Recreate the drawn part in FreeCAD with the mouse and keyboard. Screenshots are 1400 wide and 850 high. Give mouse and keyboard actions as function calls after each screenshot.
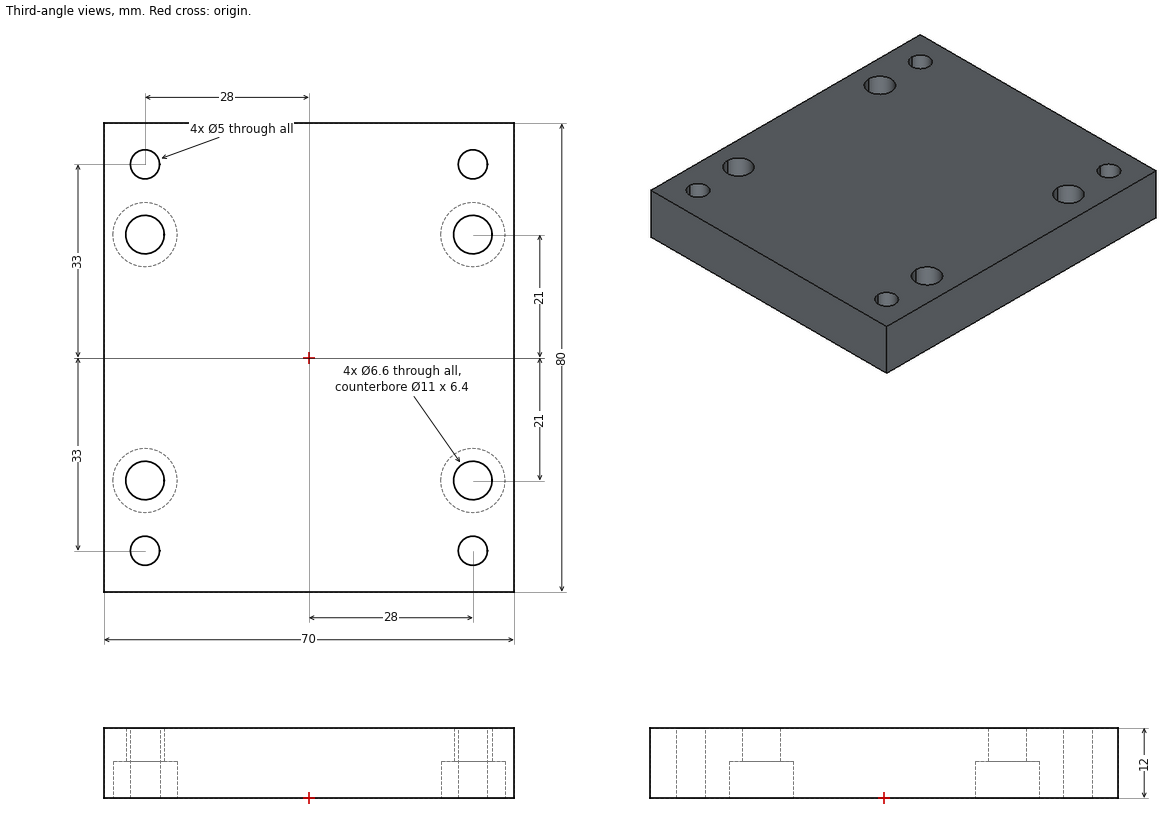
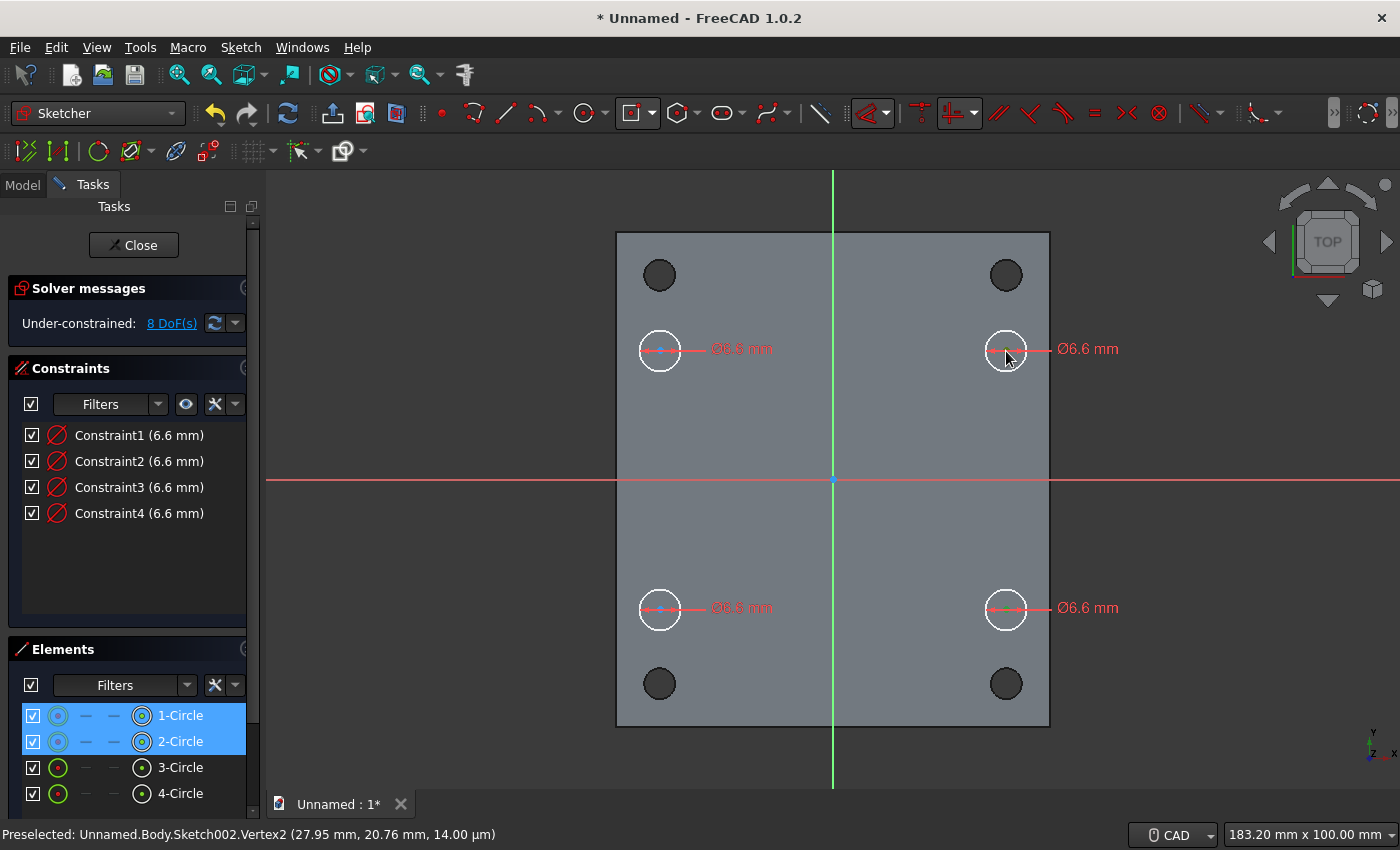
click(976, 114)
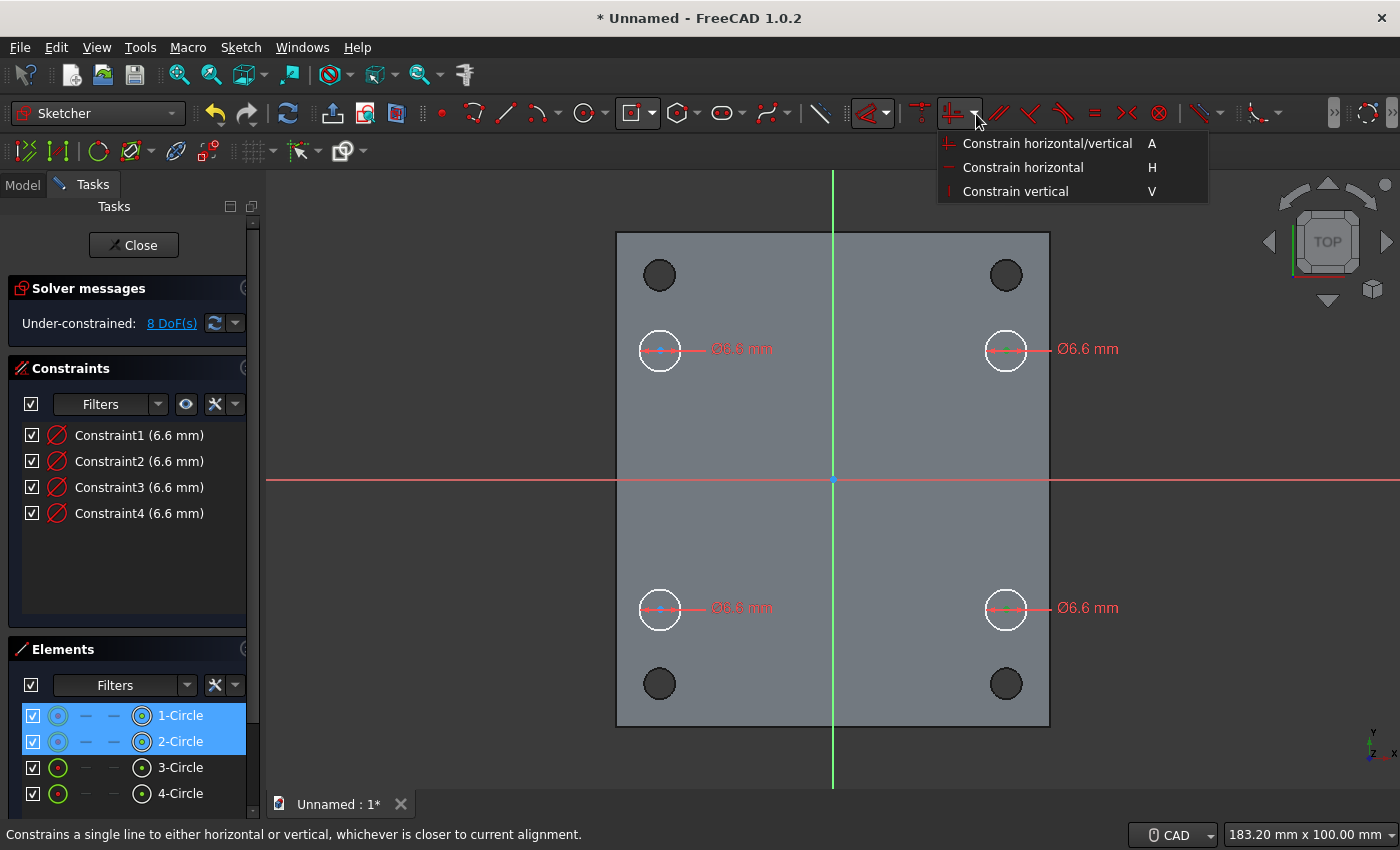
click(1073, 191)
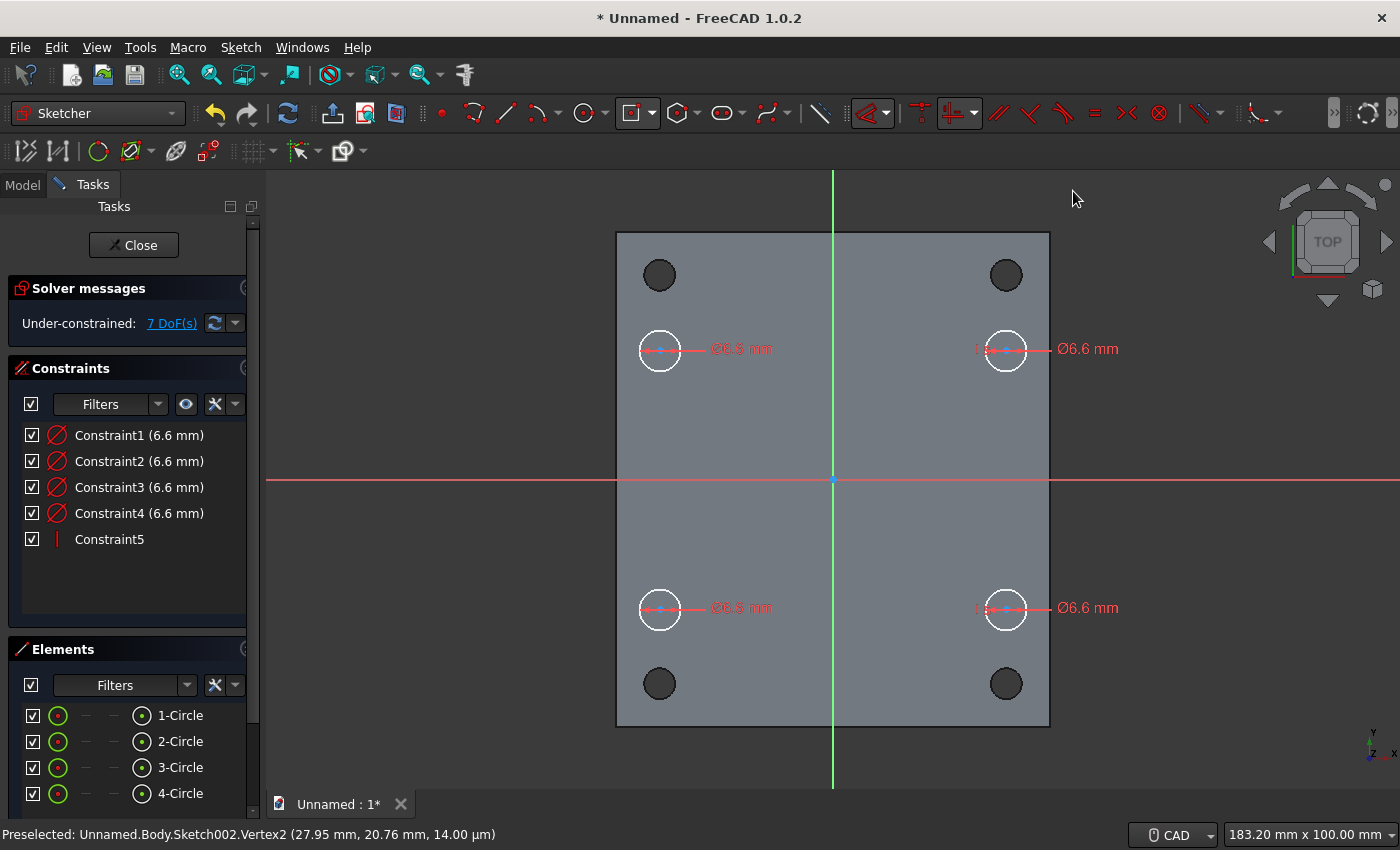
click(1006, 610)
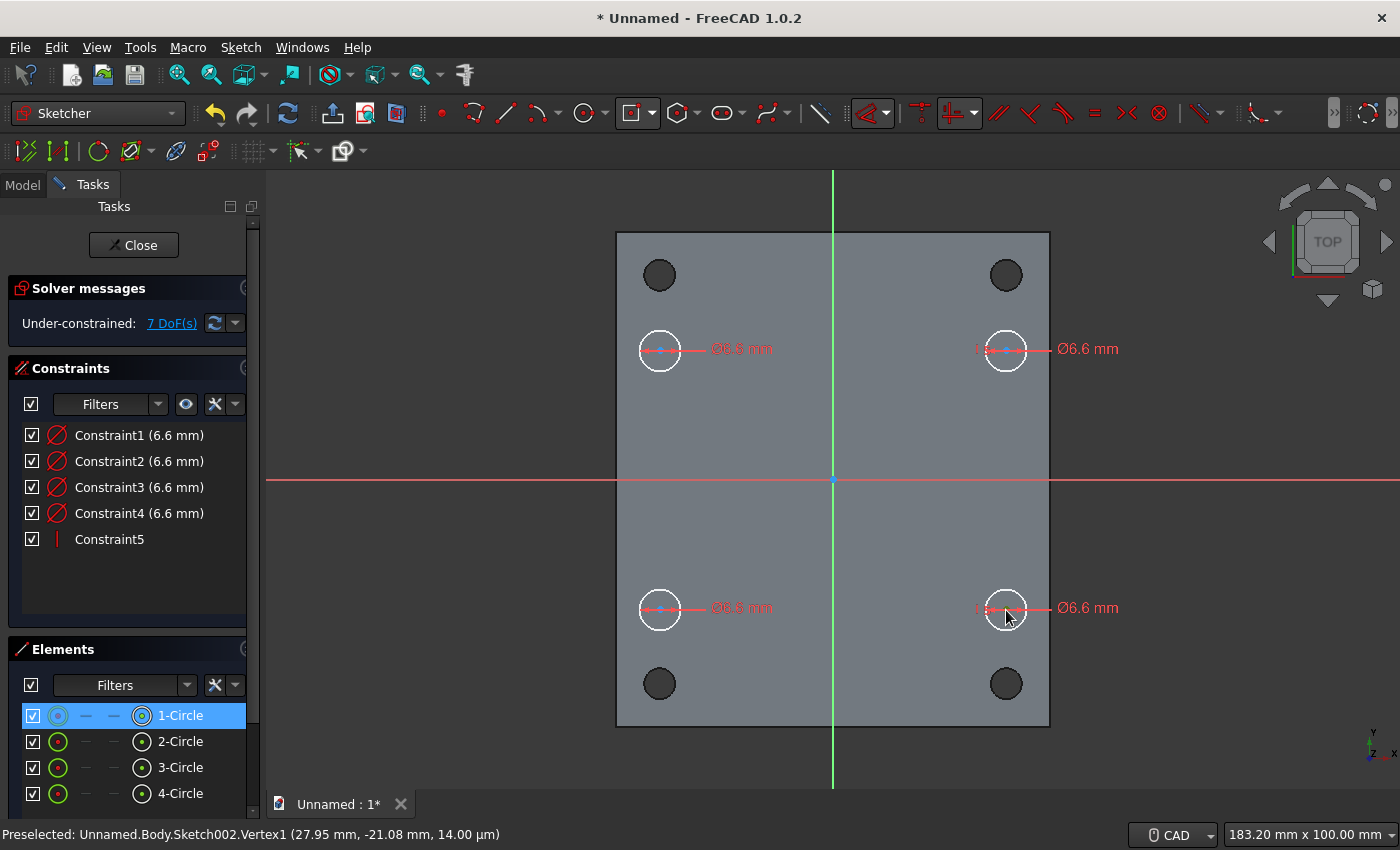
click(660, 610)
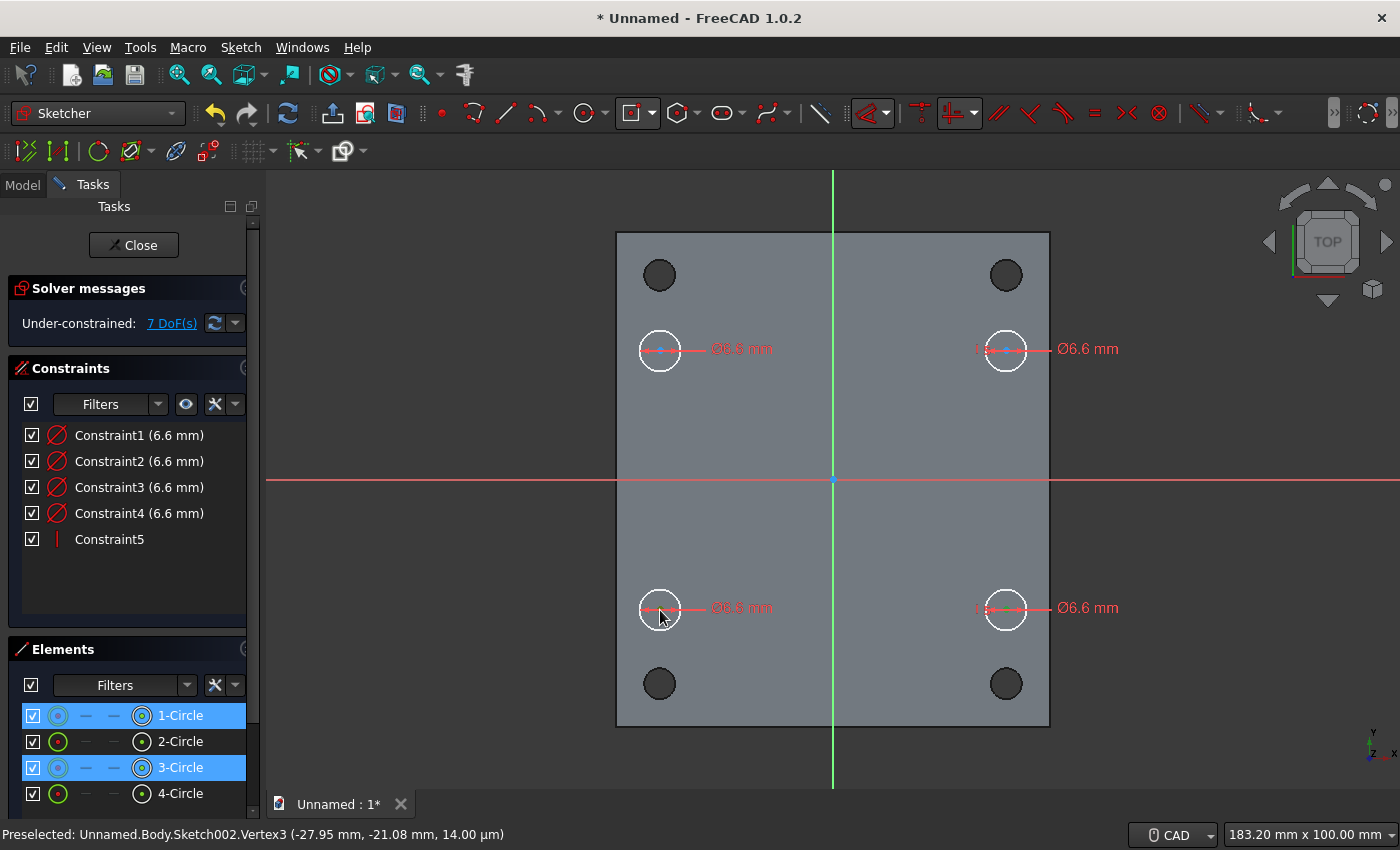
click(976, 114)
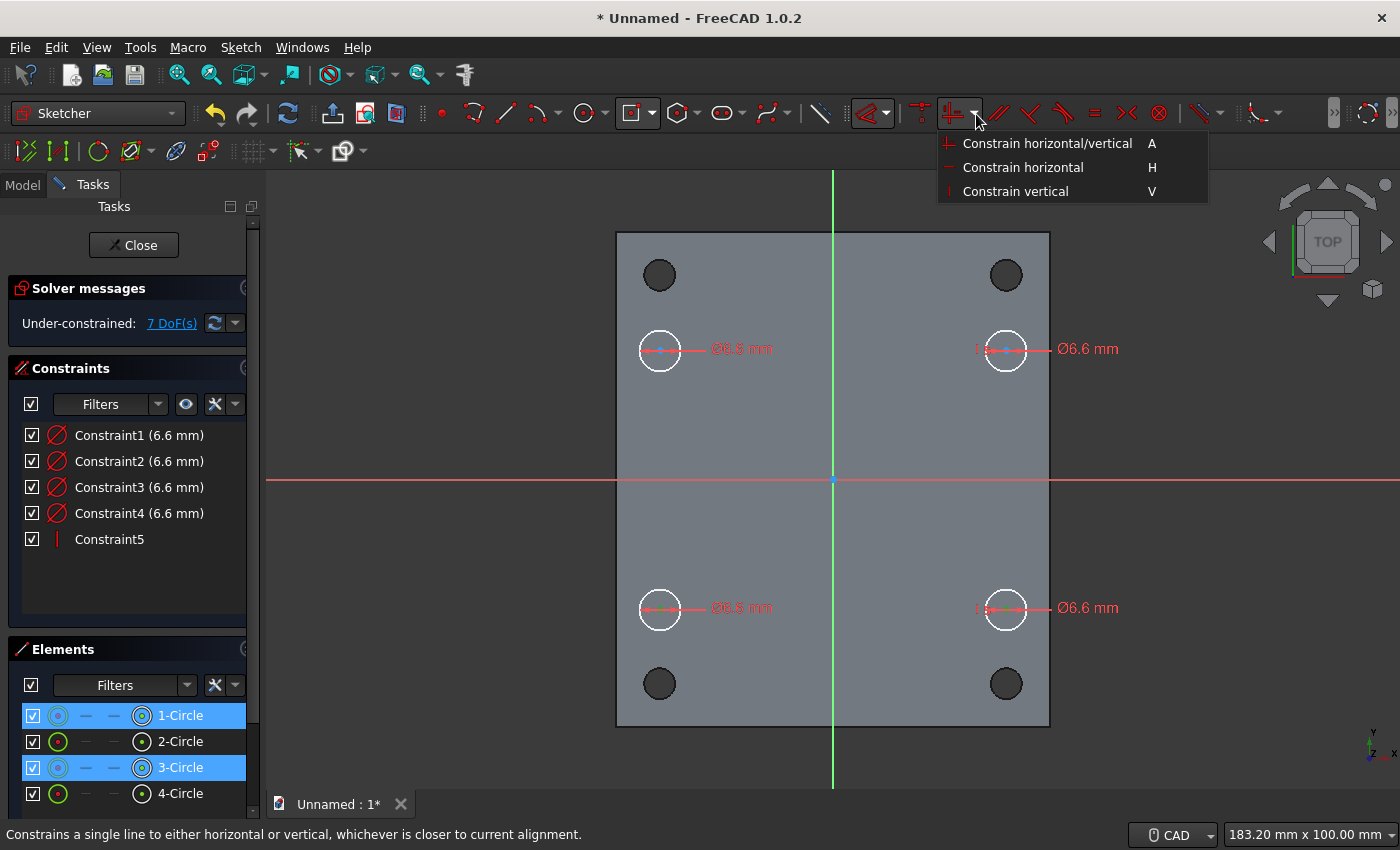
click(1073, 167)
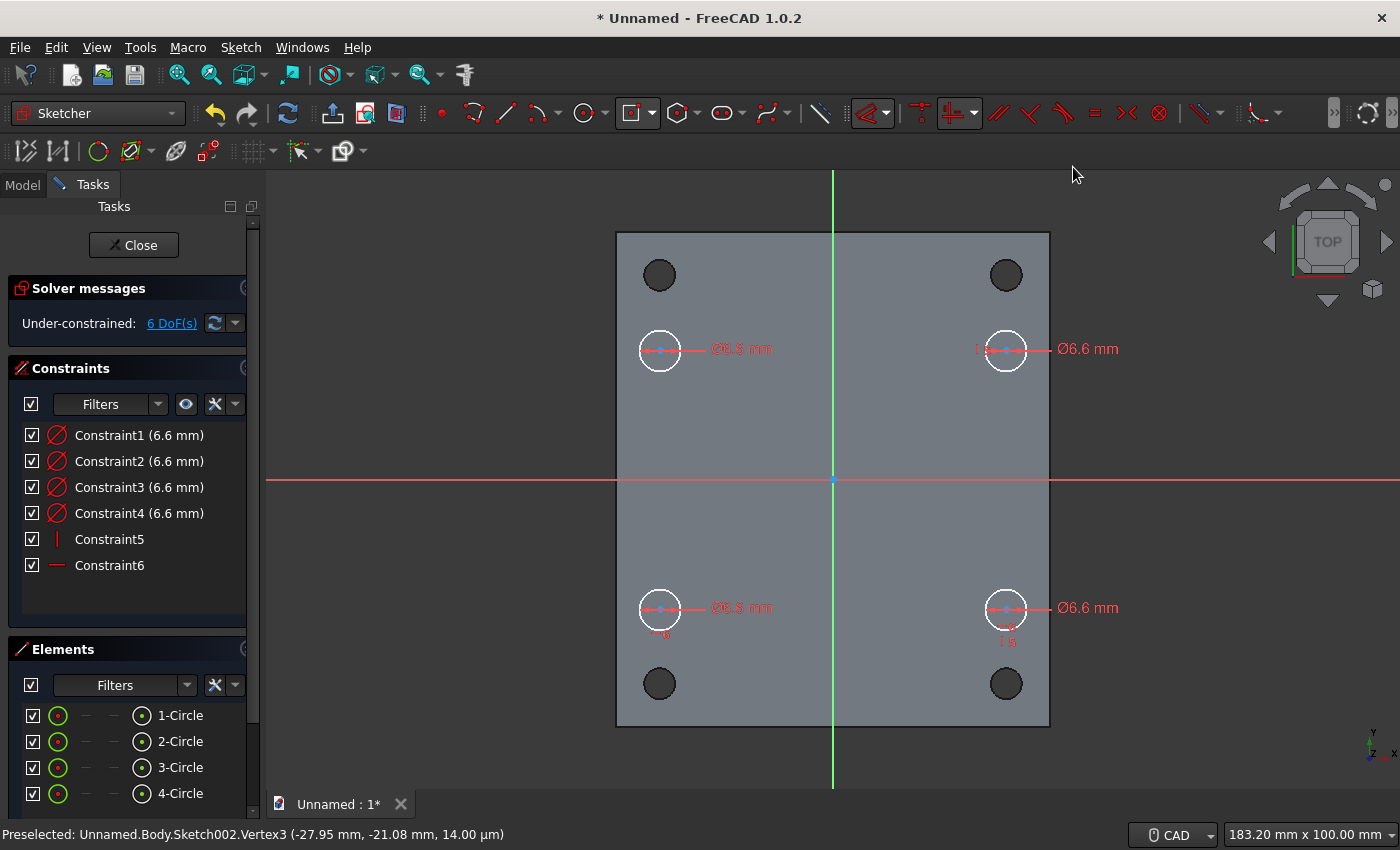
click(660, 610)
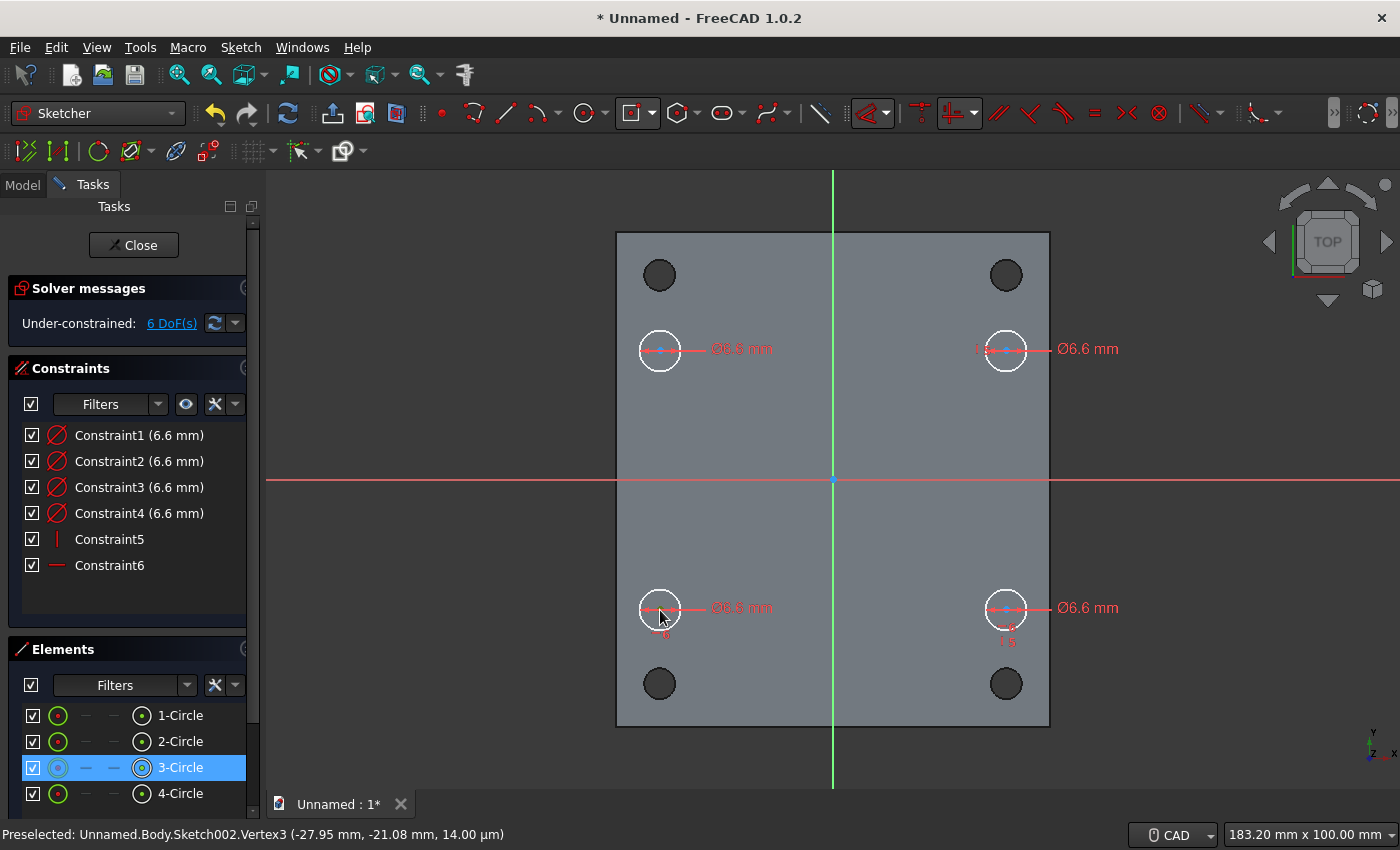
click(660, 351)